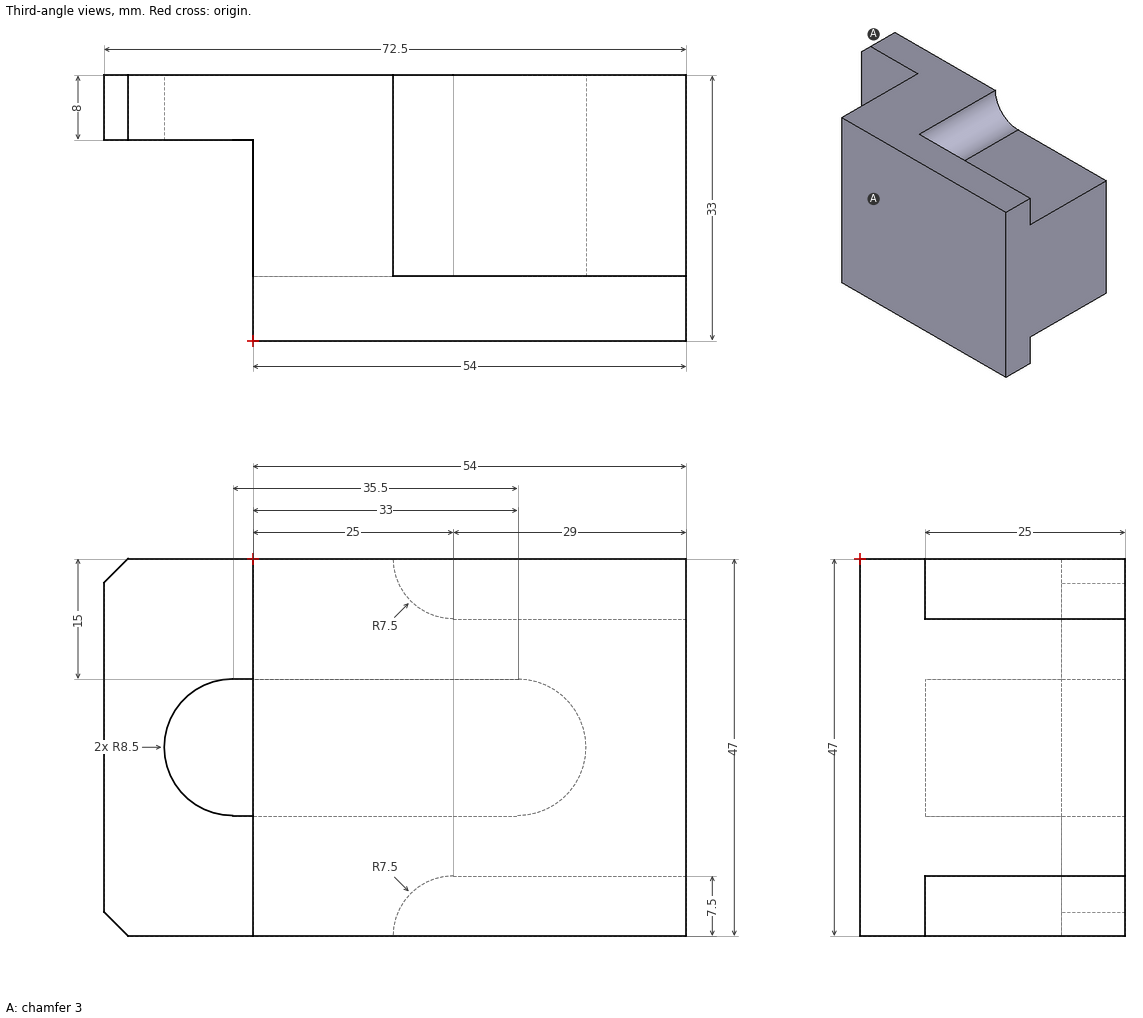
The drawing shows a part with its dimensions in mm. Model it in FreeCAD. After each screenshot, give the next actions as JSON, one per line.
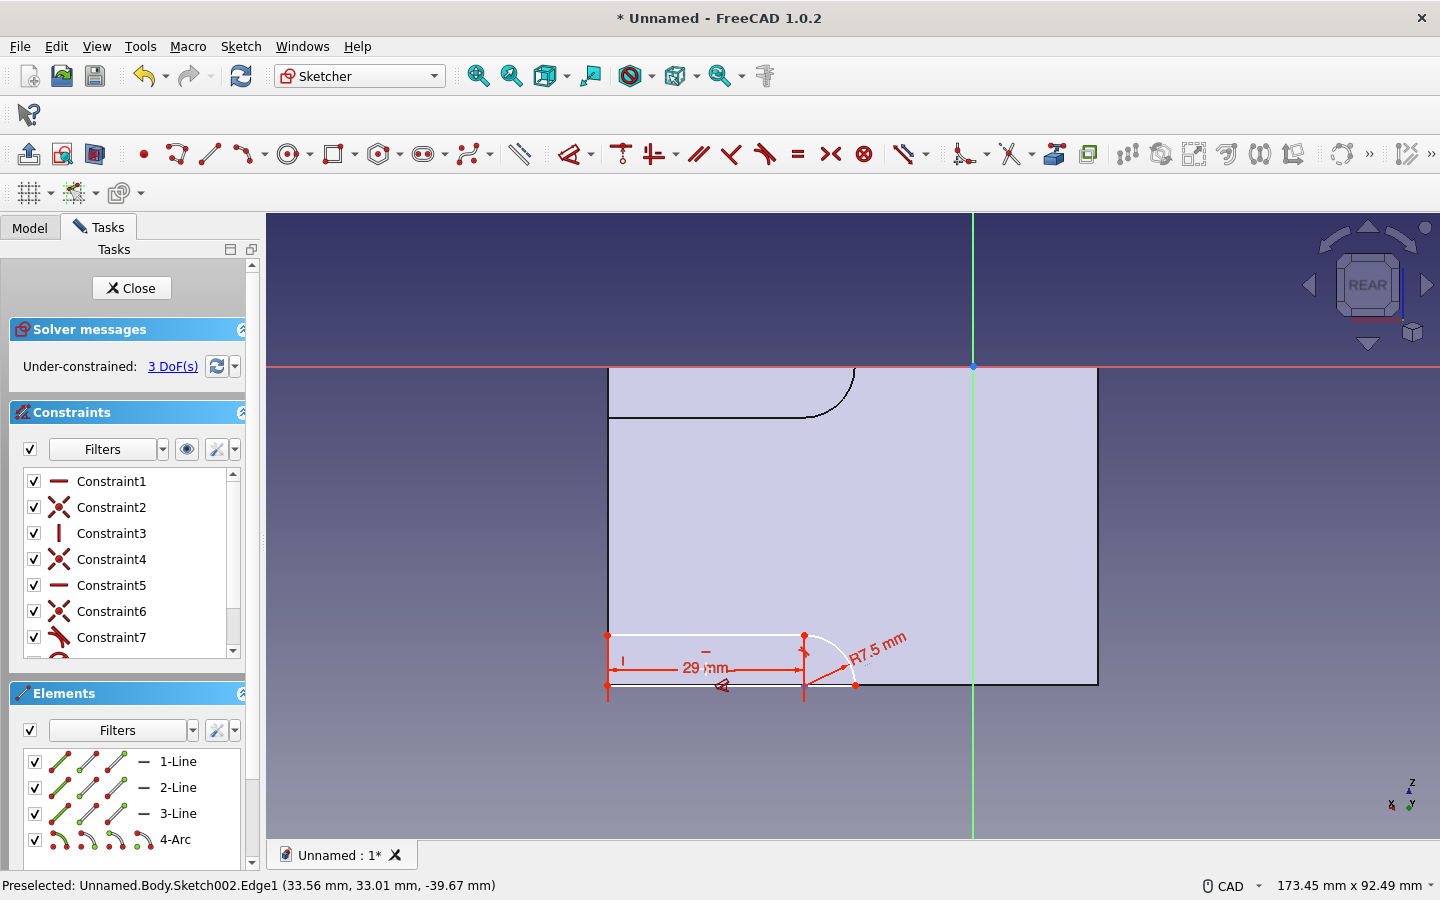
{"action": "left_click", "coordinate": [608, 651]}
{"action": "left_click", "coordinate": [574, 661]}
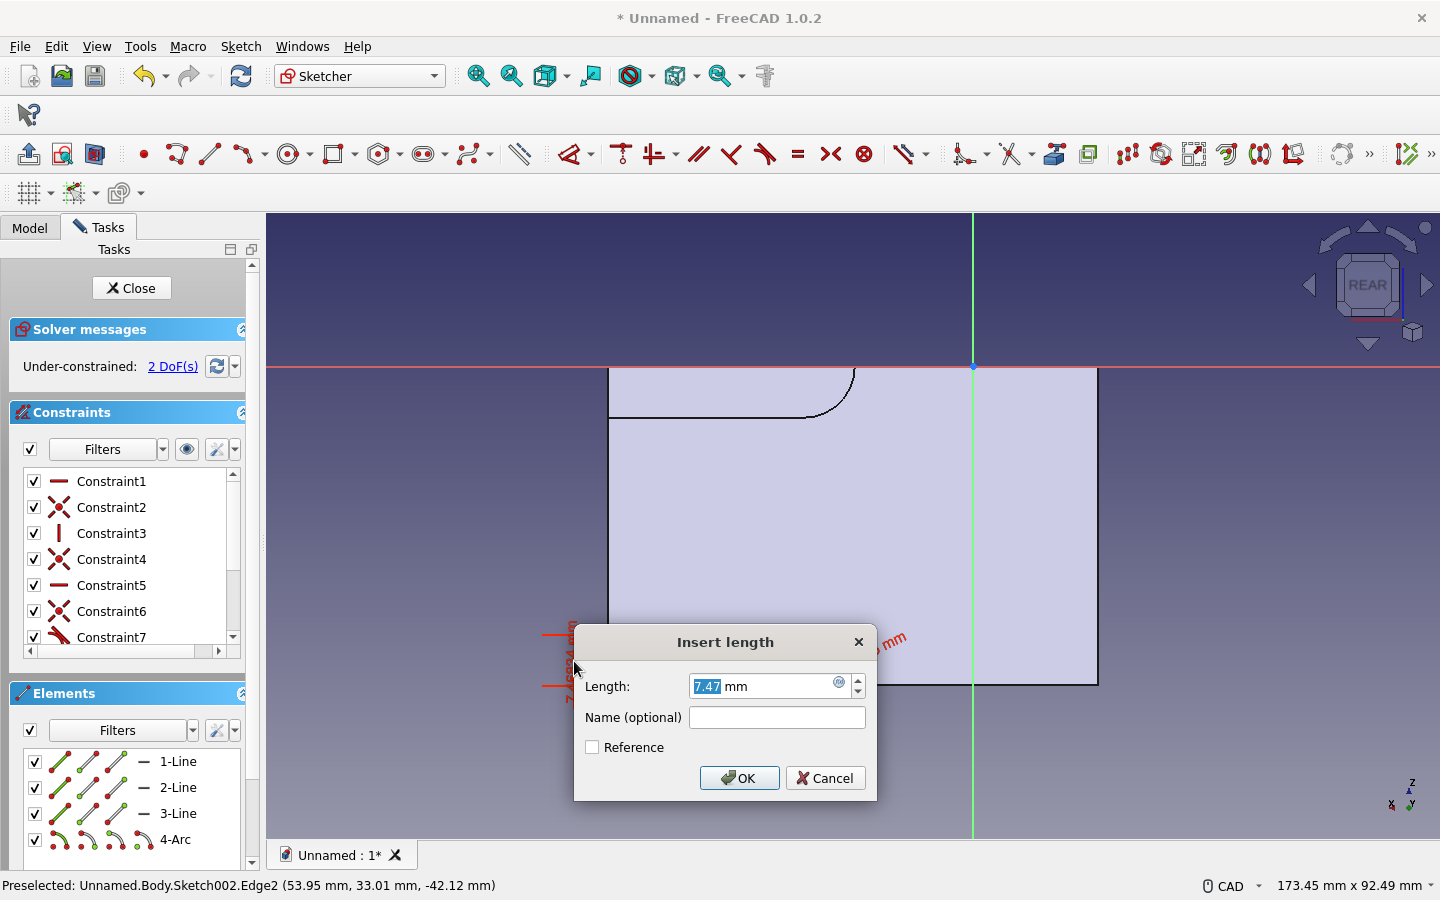
{"action": "type", "text": "7.5"}
{"action": "key", "text": "Return"}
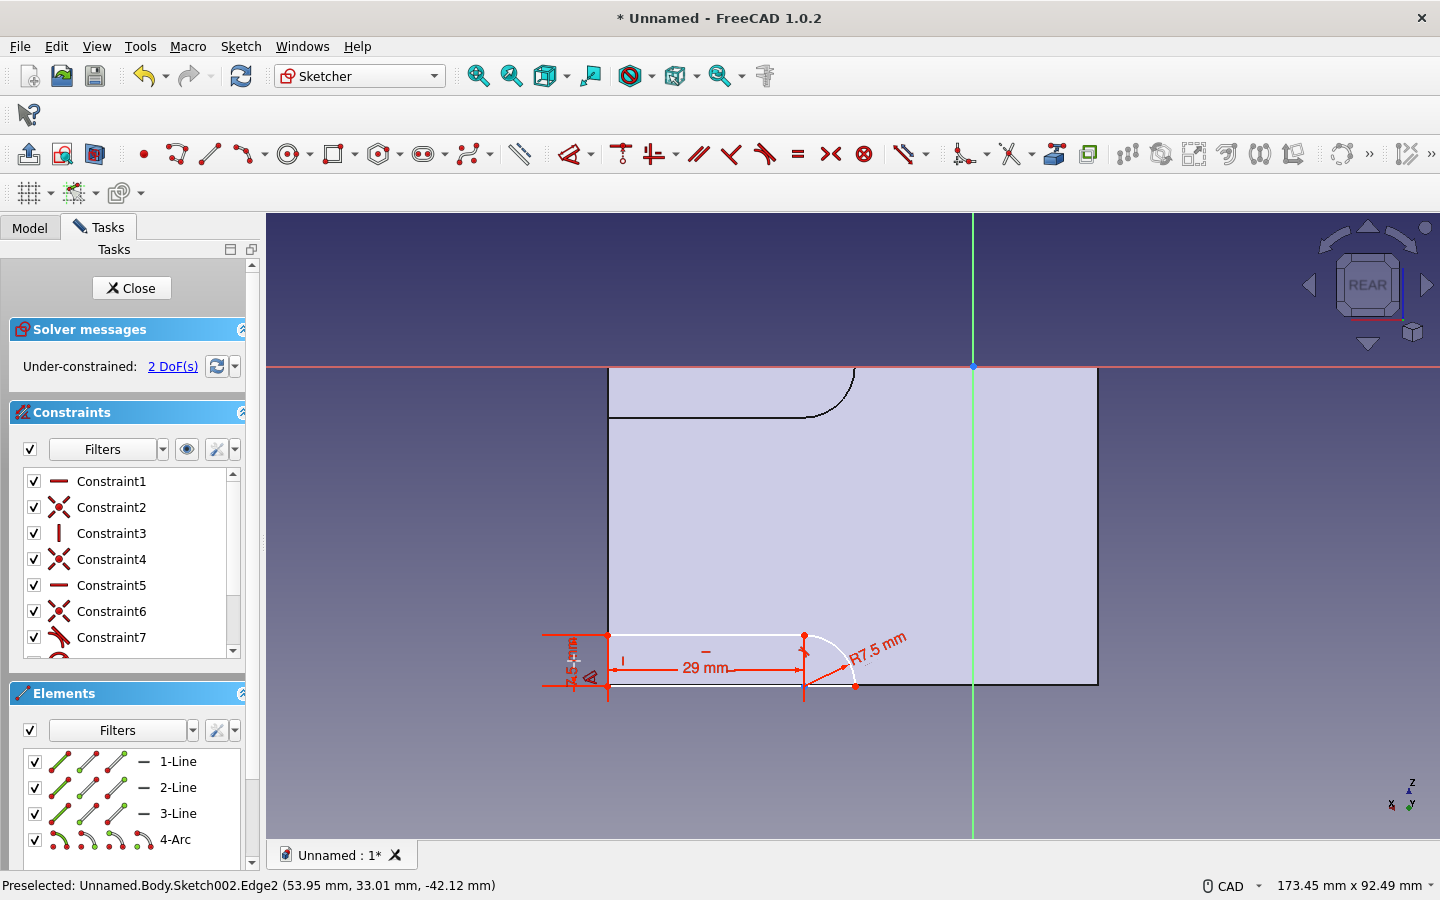
{"action": "left_click", "coordinate": [804, 635]}
{"action": "left_click", "coordinate": [889, 333]}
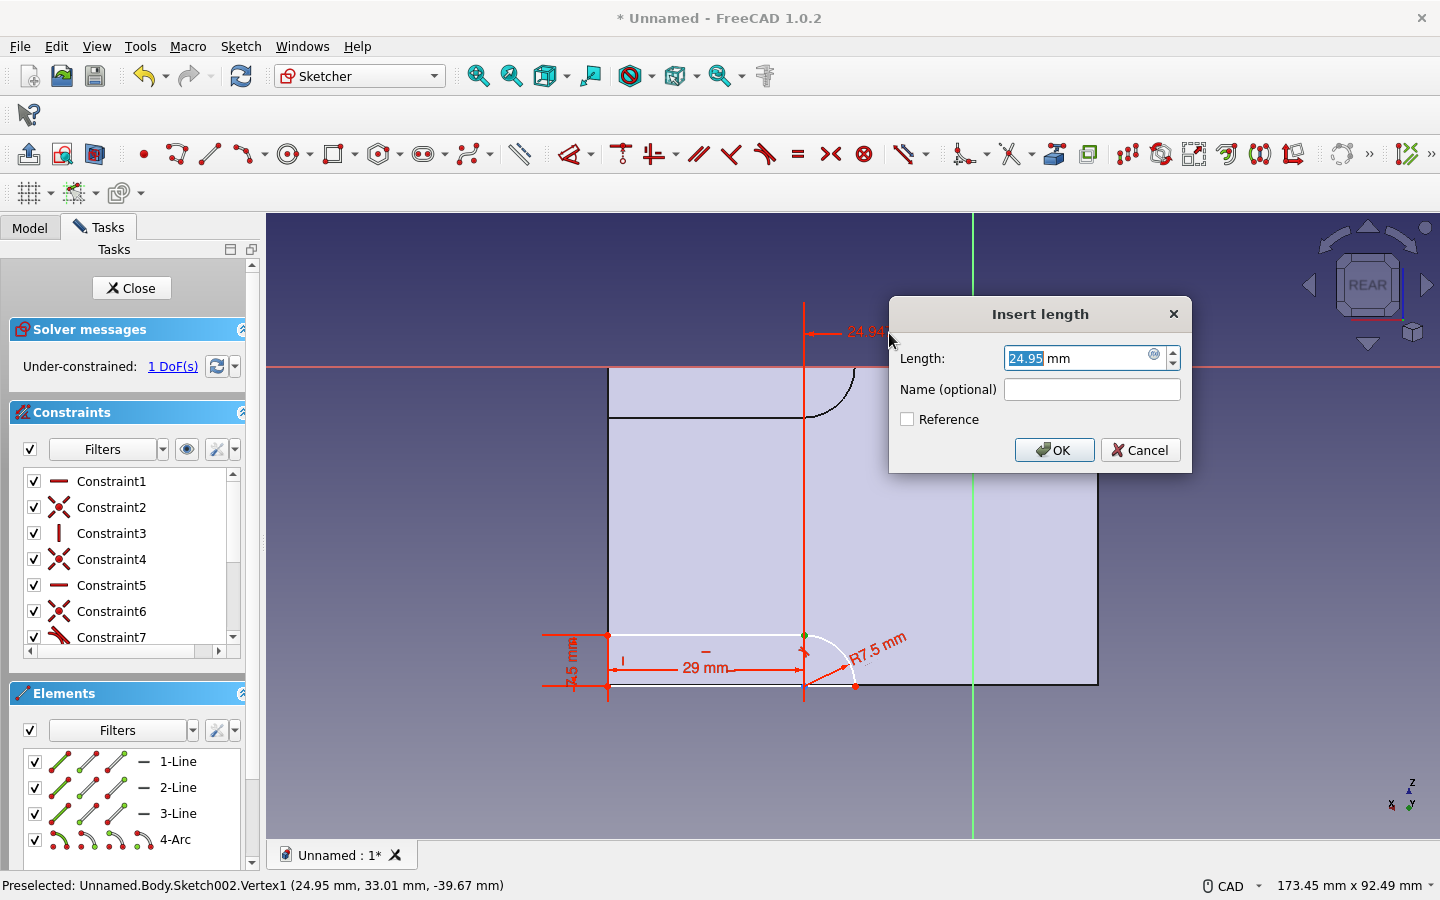
{"action": "type", "text": "25"}
{"action": "key", "text": "Return"}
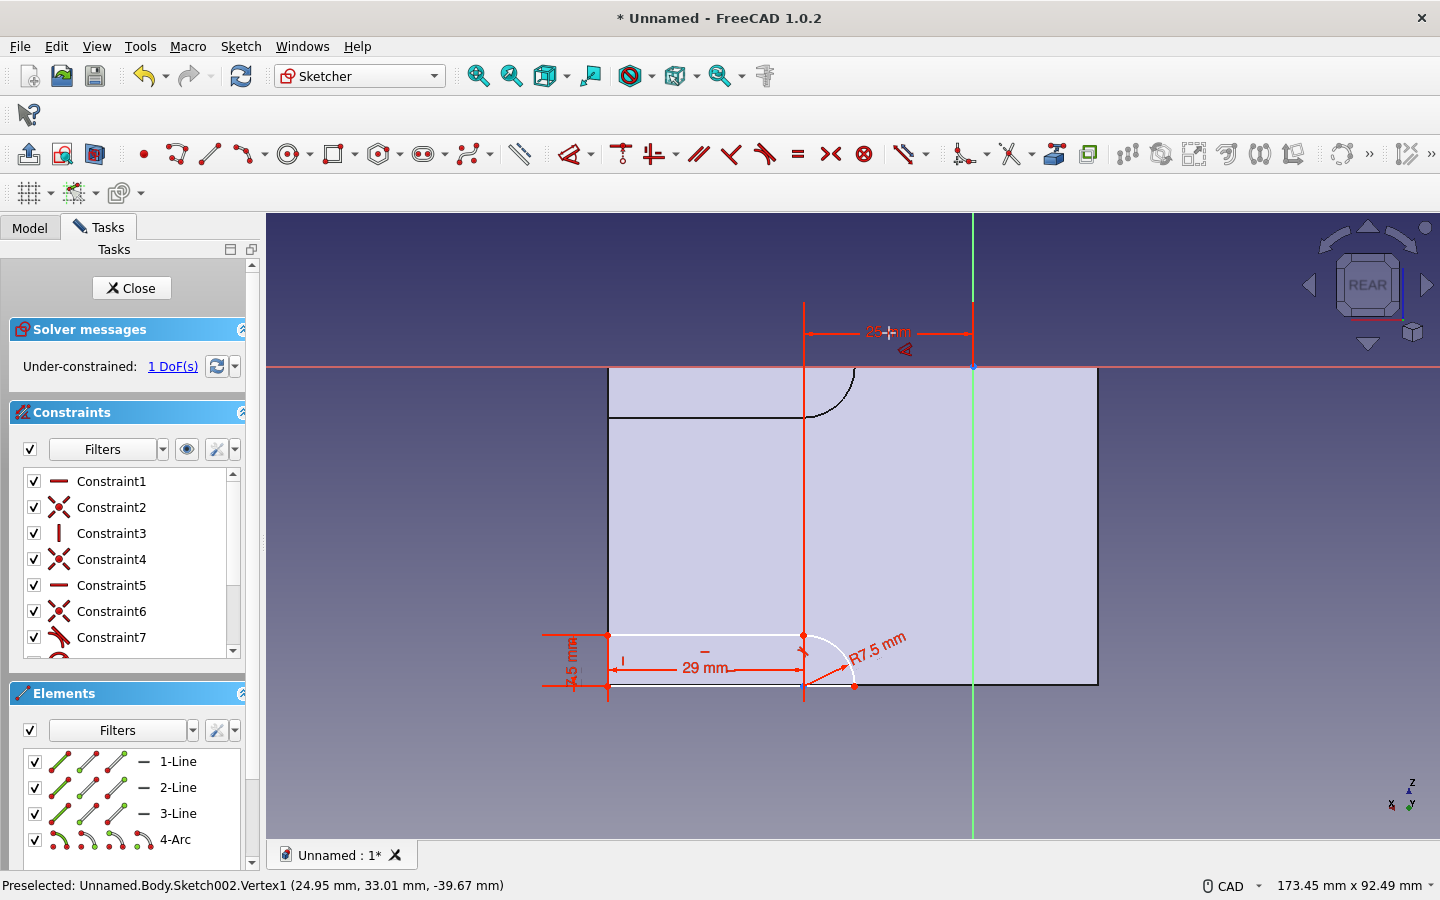
{"action": "left_click", "coordinate": [608, 686]}
{"action": "left_click", "coordinate": [1007, 527]}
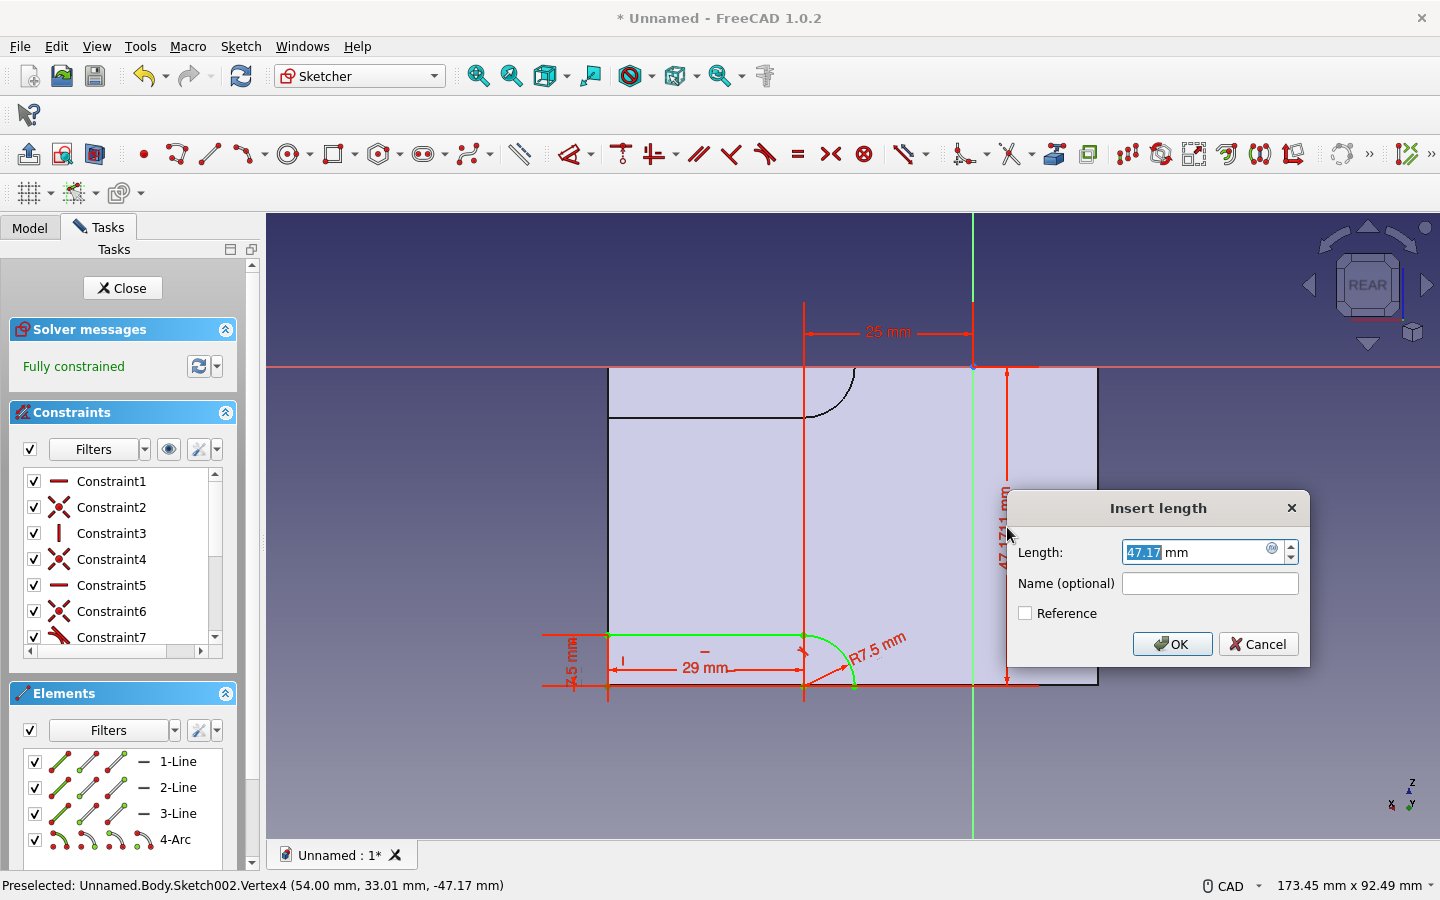
{"action": "type", "text": "47"}
{"action": "key", "text": "Return"}
{"action": "key", "text": "Escape"}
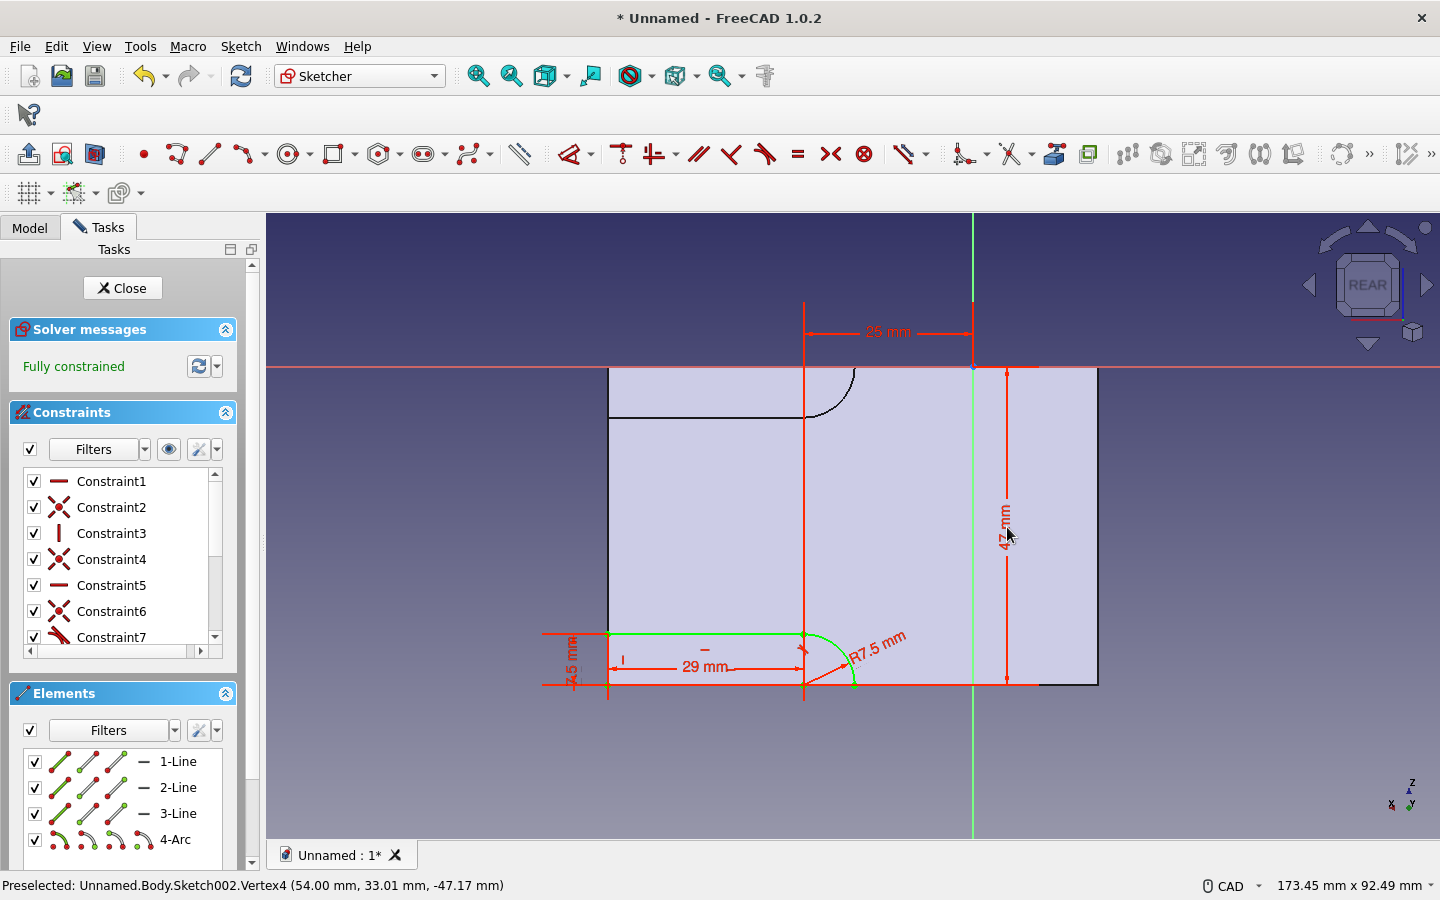
{"action": "left_click", "coordinate": [123, 288]}